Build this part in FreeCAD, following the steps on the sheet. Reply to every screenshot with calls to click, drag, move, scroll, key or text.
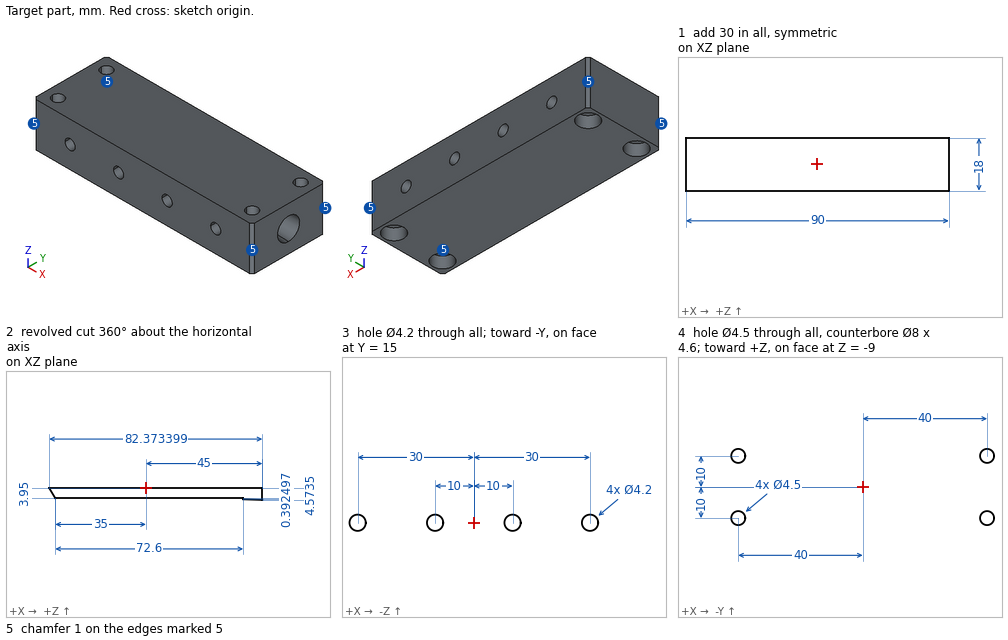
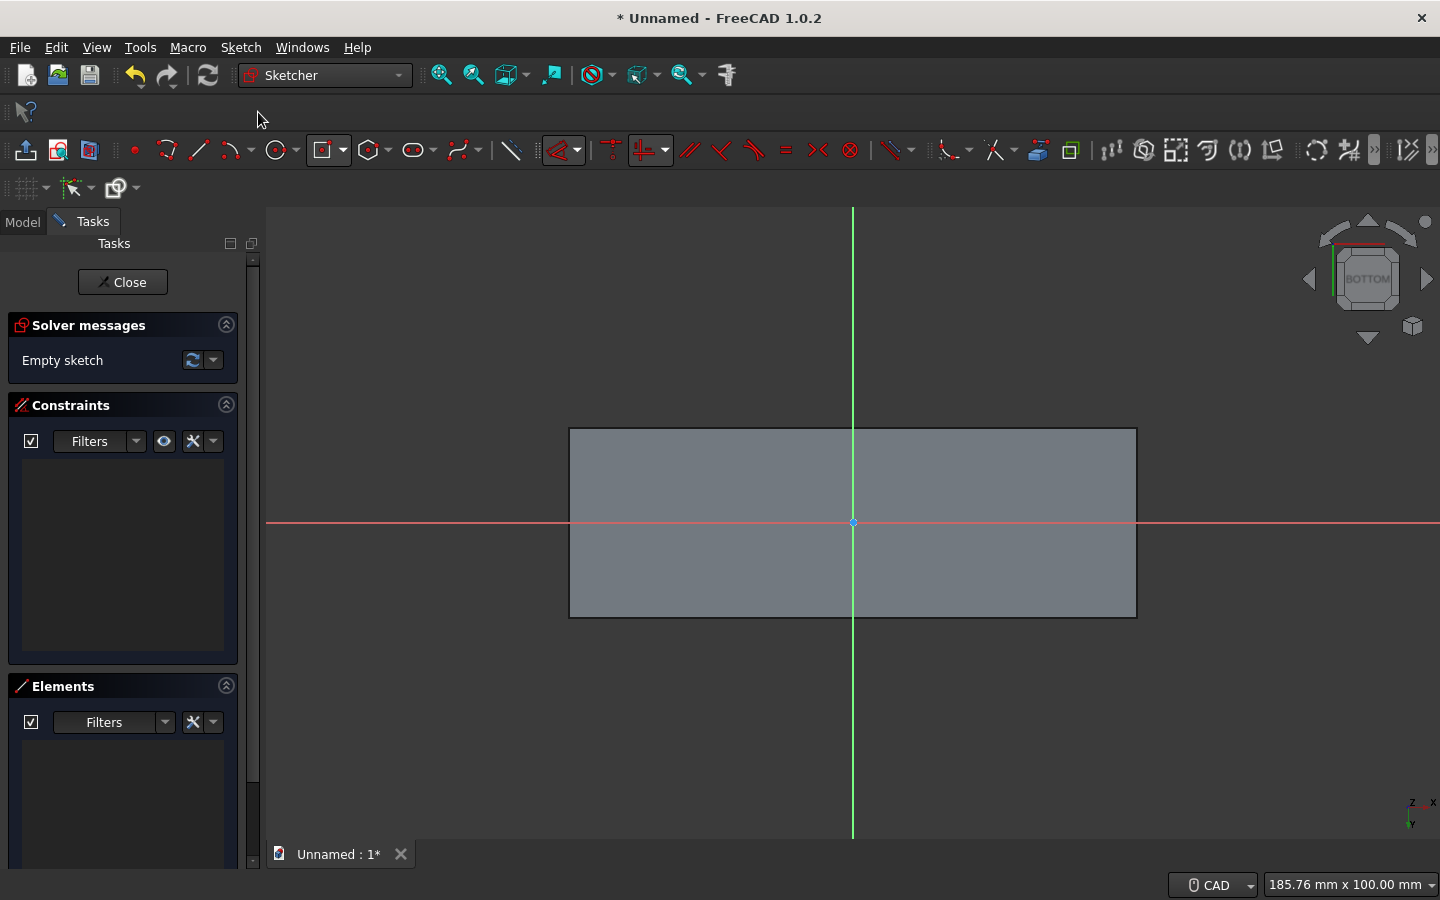
click(276, 150)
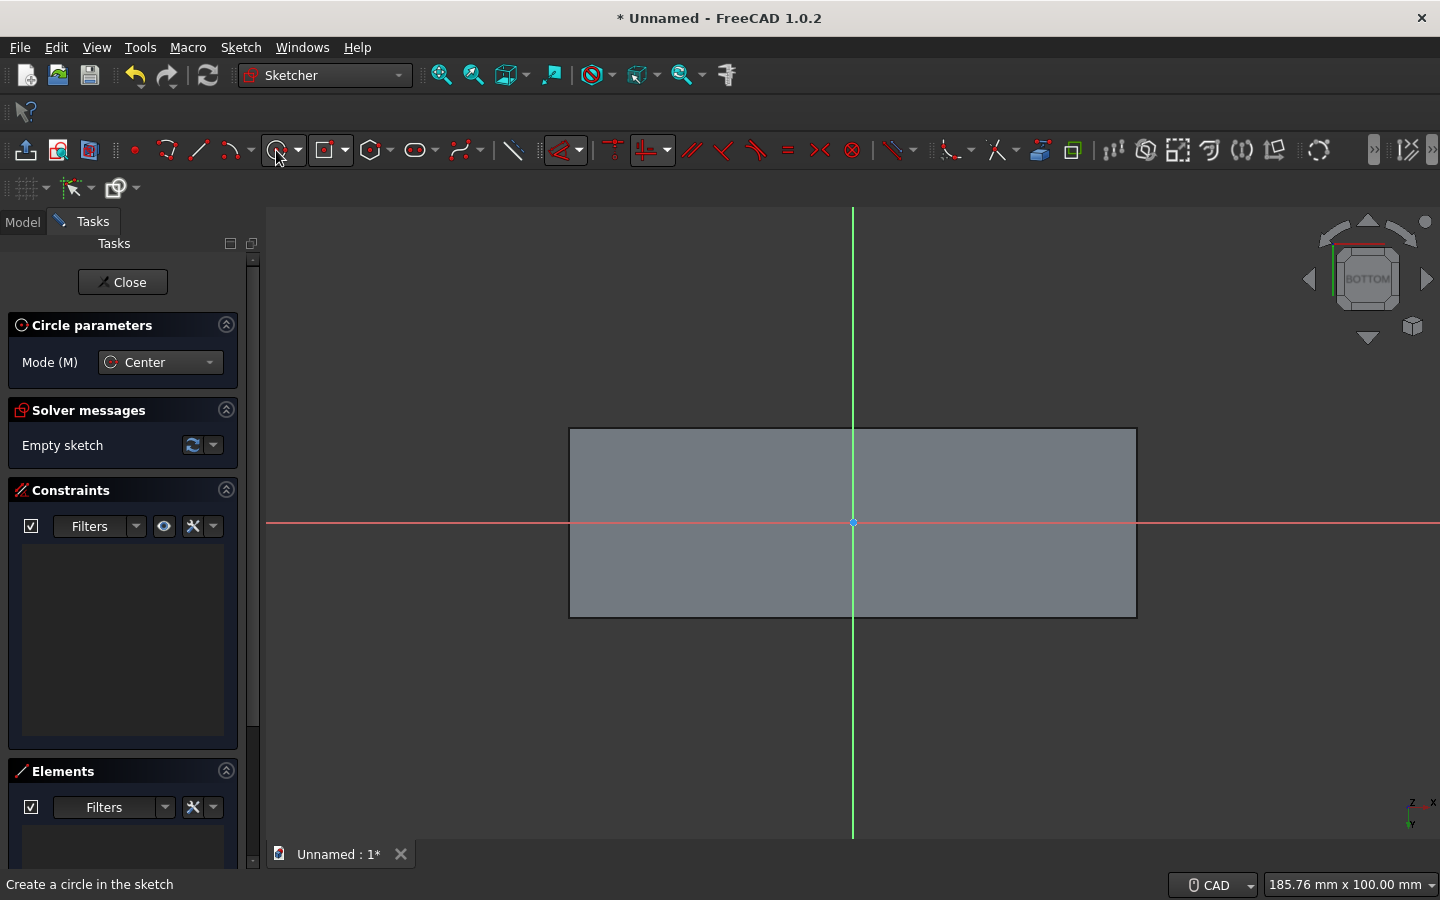
scroll(600, 586, up, 3)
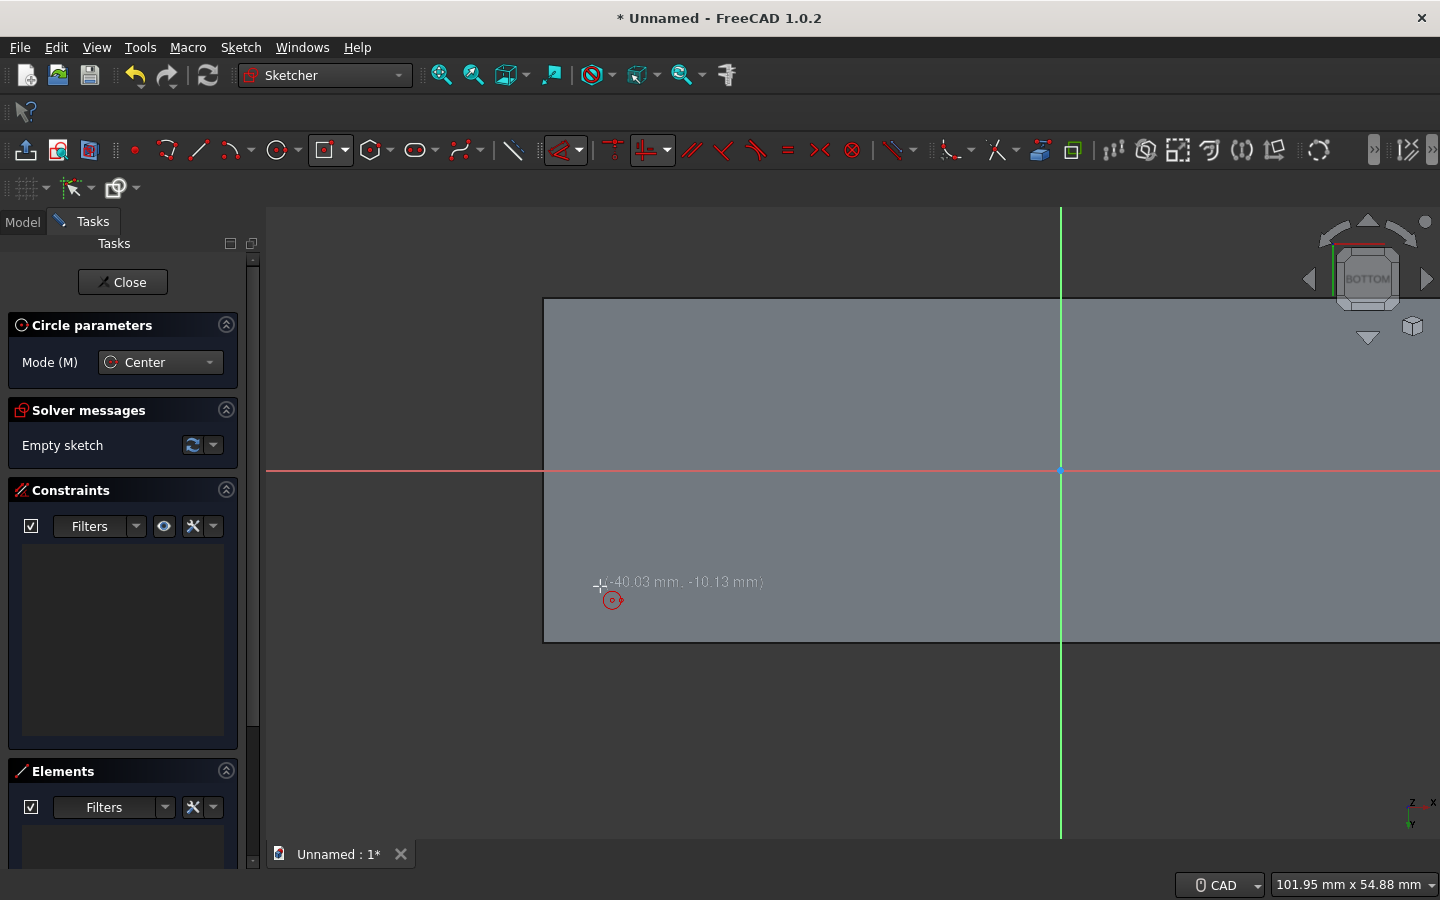
click(600, 586)
click(618, 568)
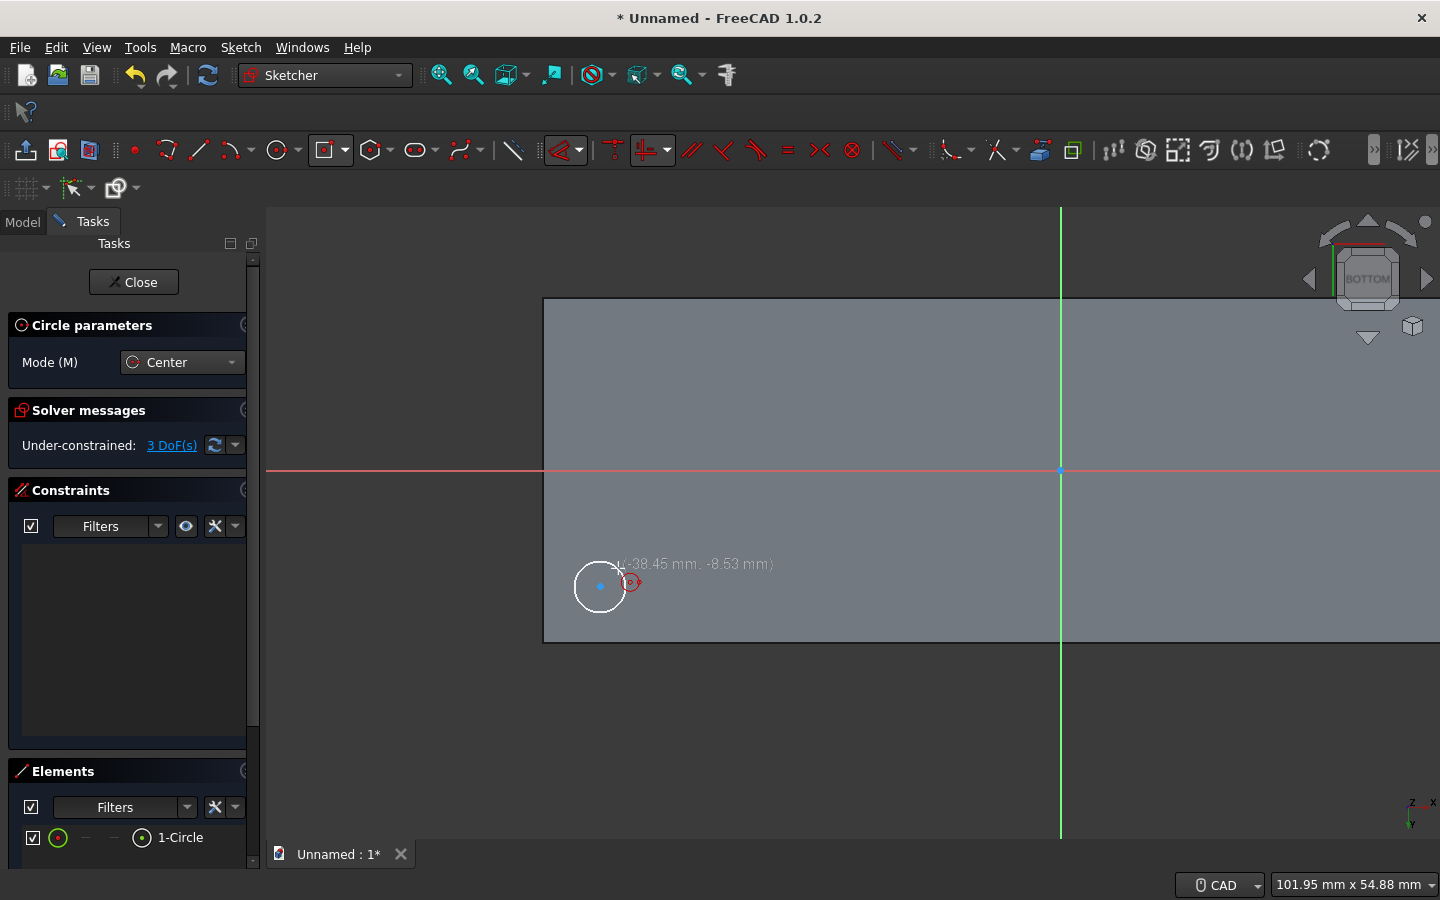
click(600, 356)
click(618, 337)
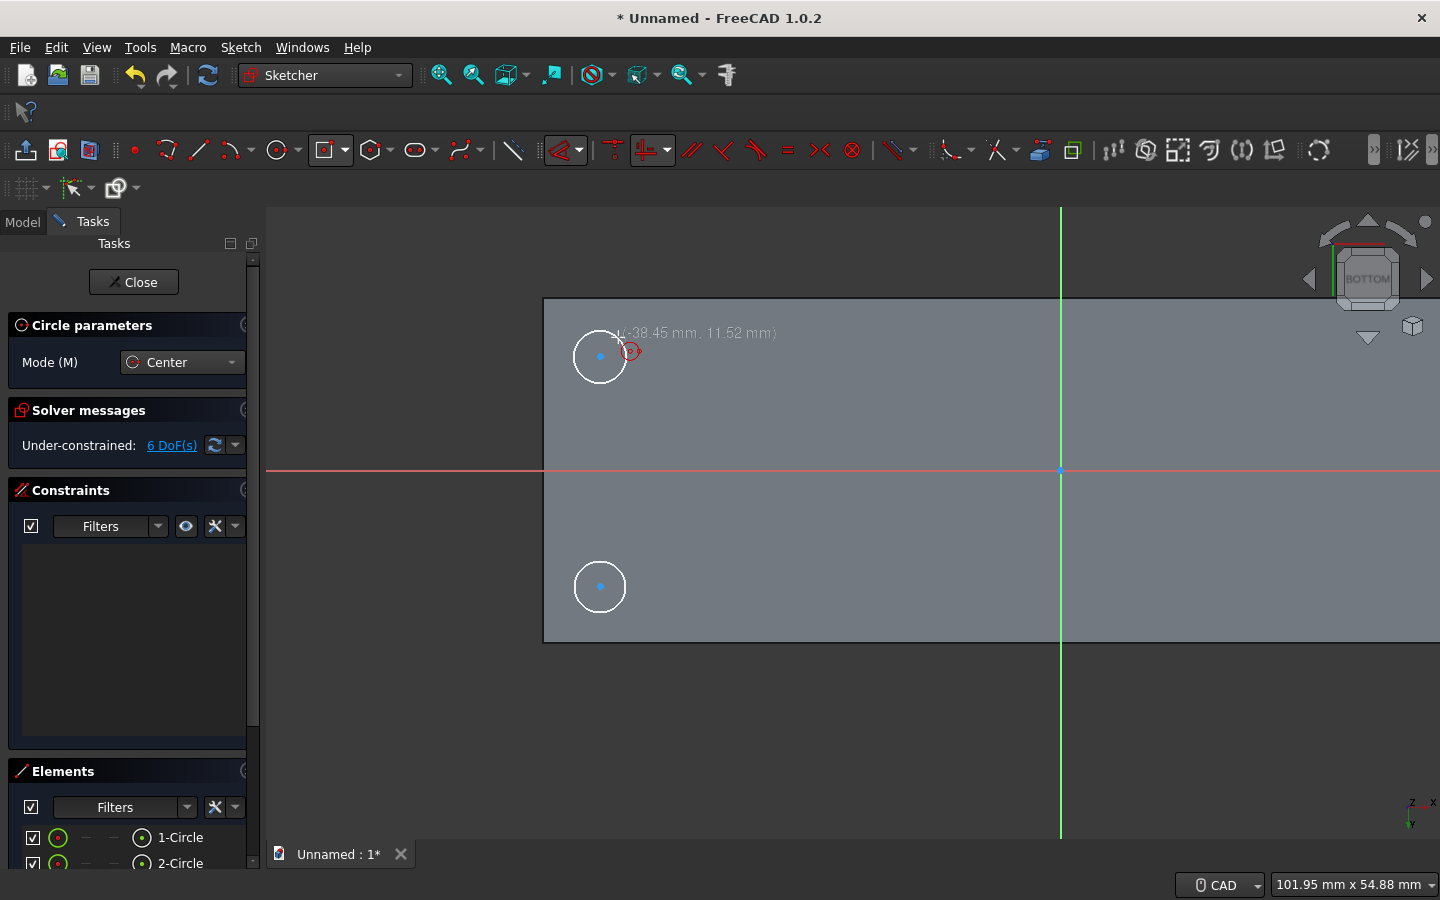
scroll(294, 629, down, 2)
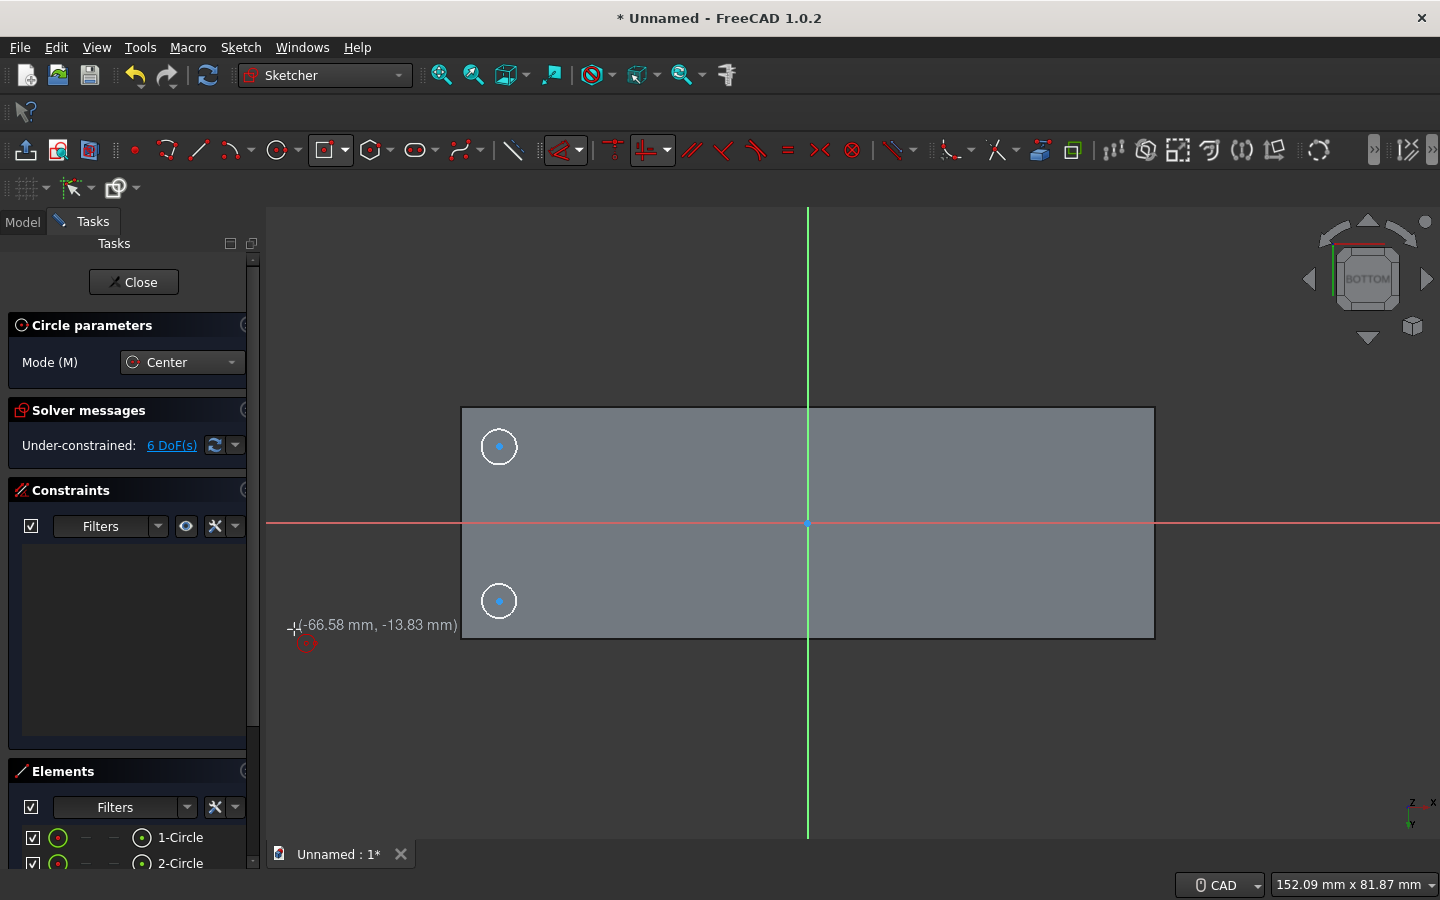
scroll(1117, 446, up, 2)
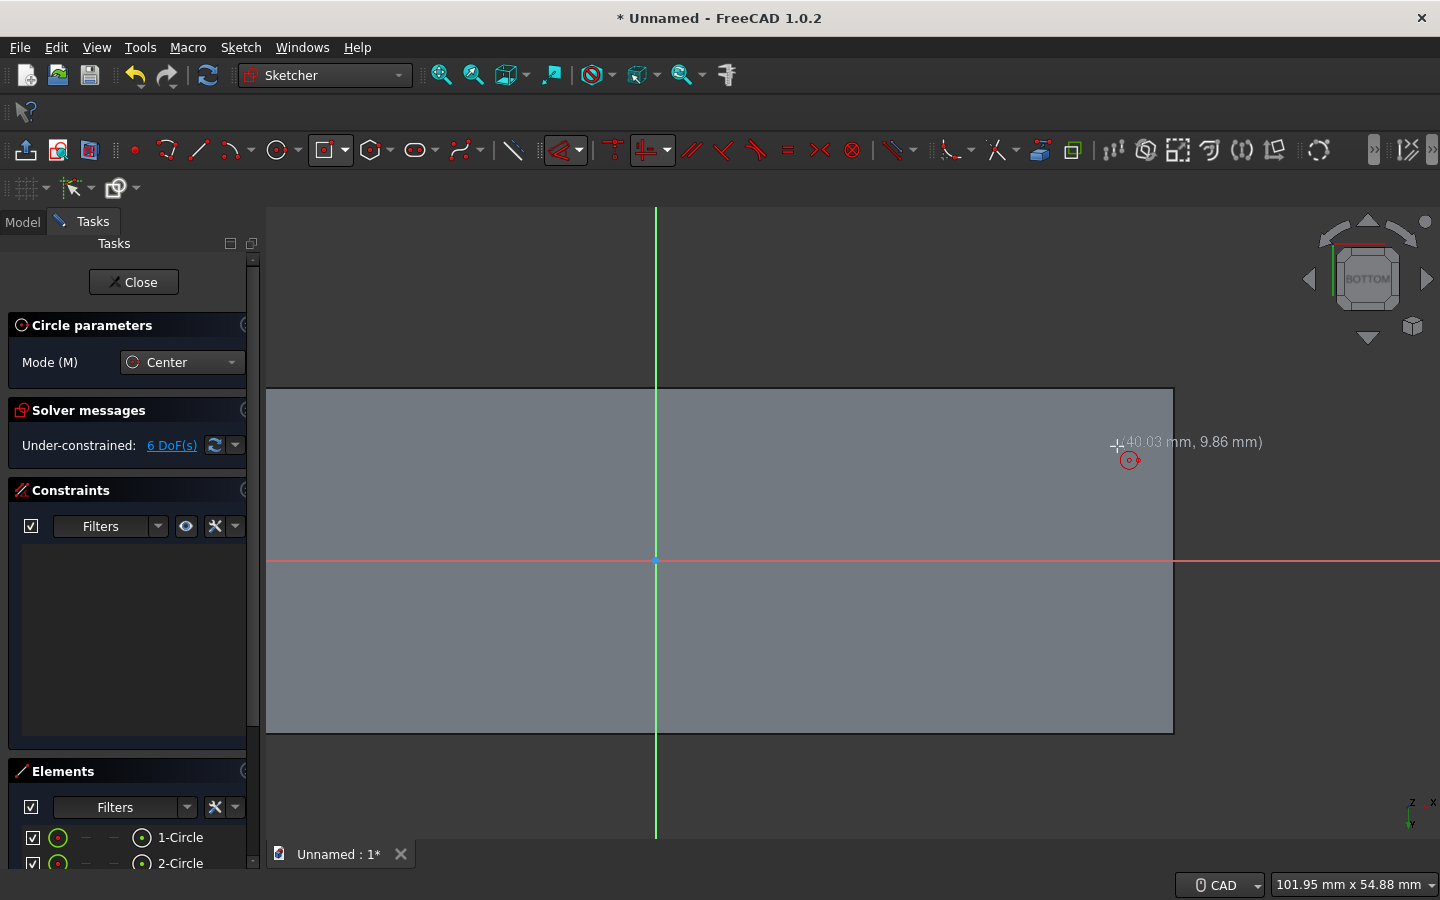
click(1116, 446)
click(1135, 427)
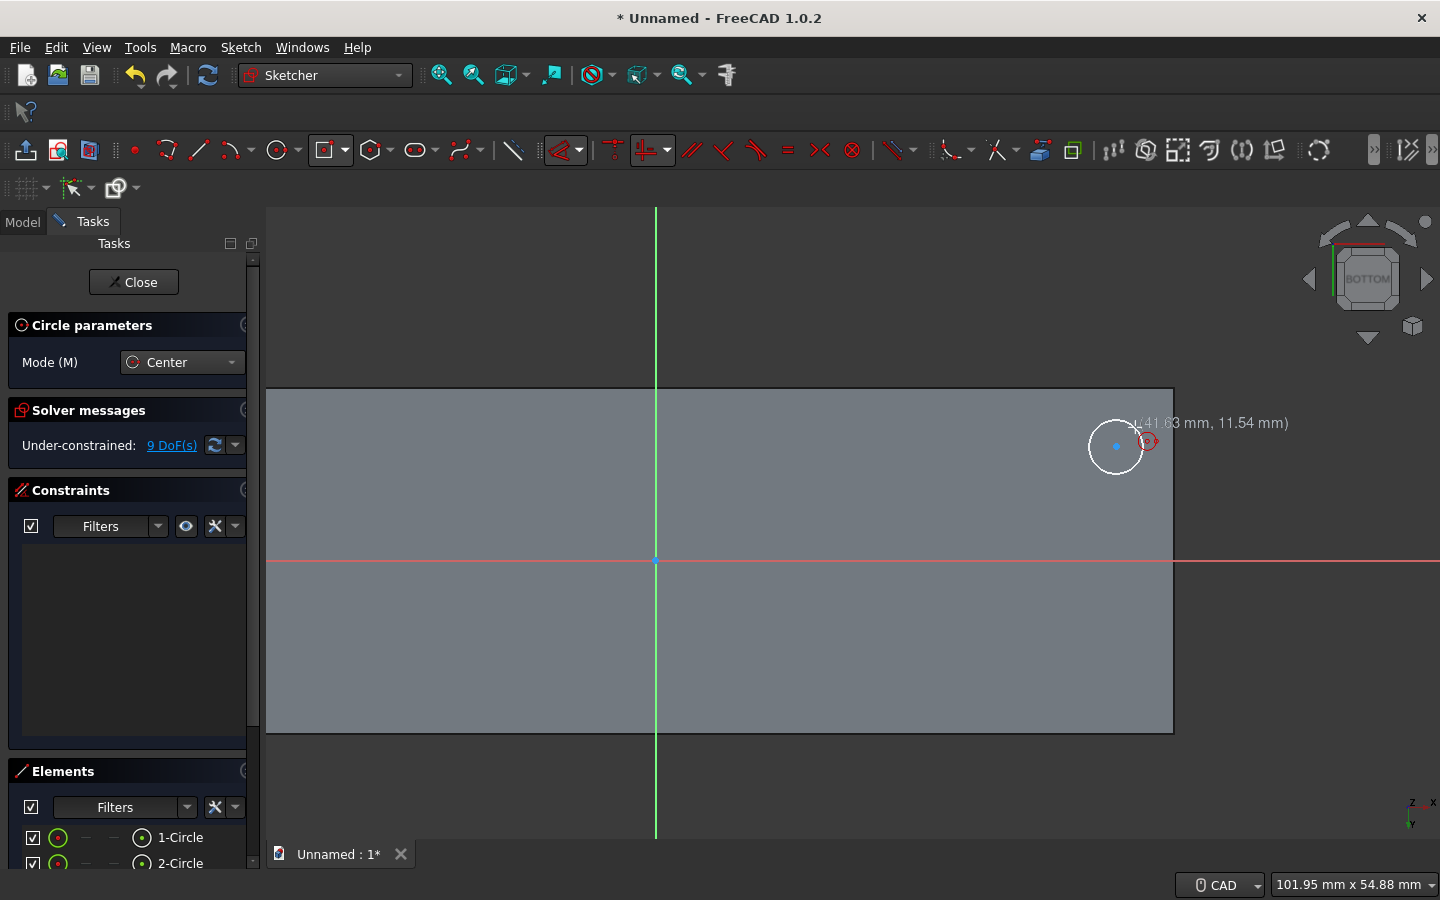
click(1116, 676)
click(1135, 658)
key(Escape)